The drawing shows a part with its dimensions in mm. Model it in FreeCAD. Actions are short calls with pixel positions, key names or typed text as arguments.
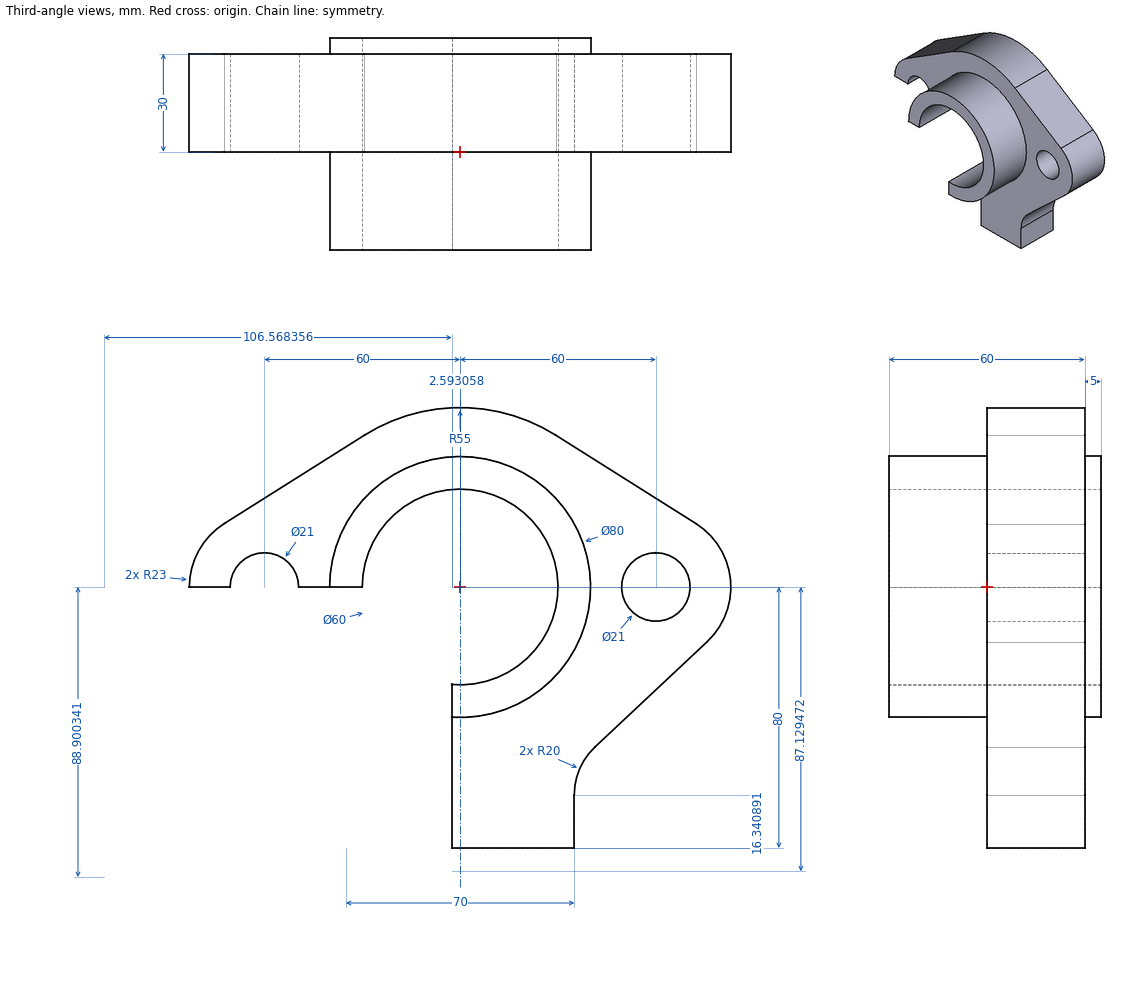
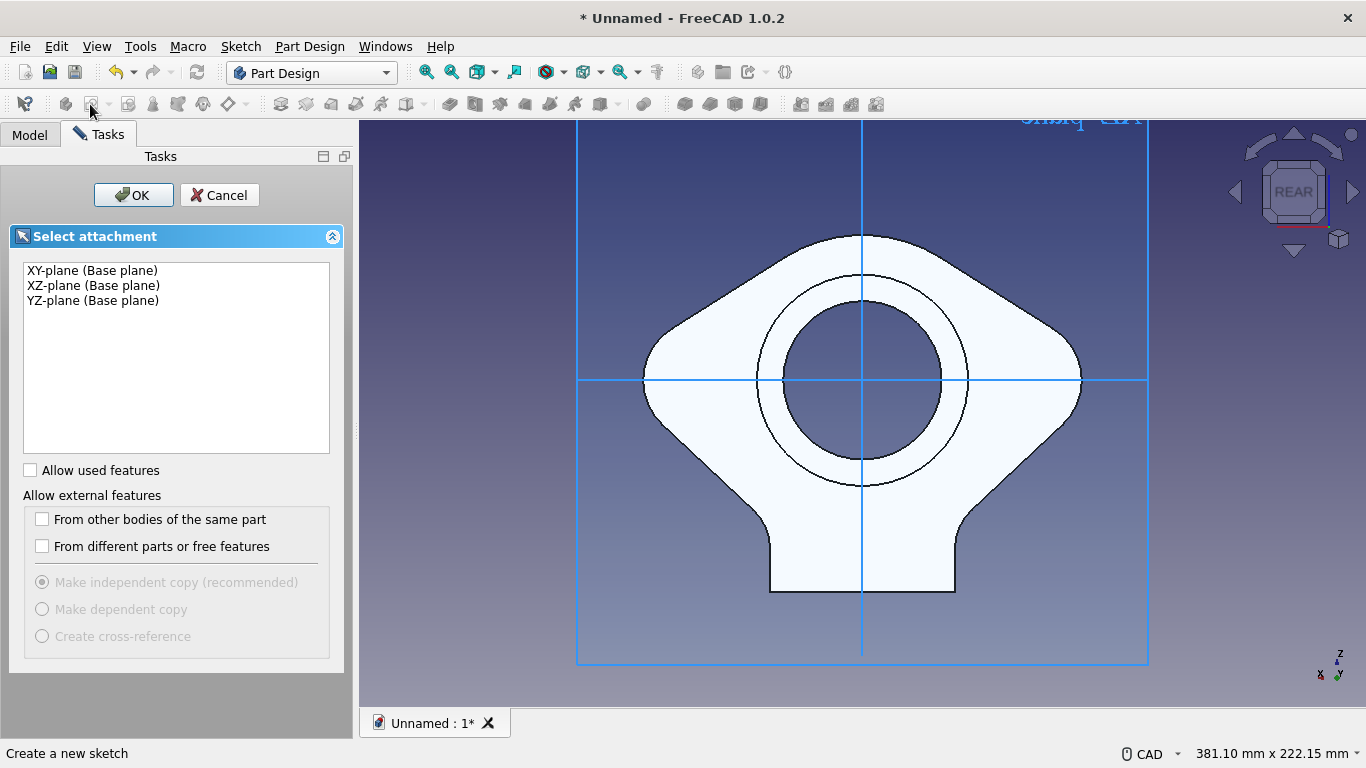
click(84, 286)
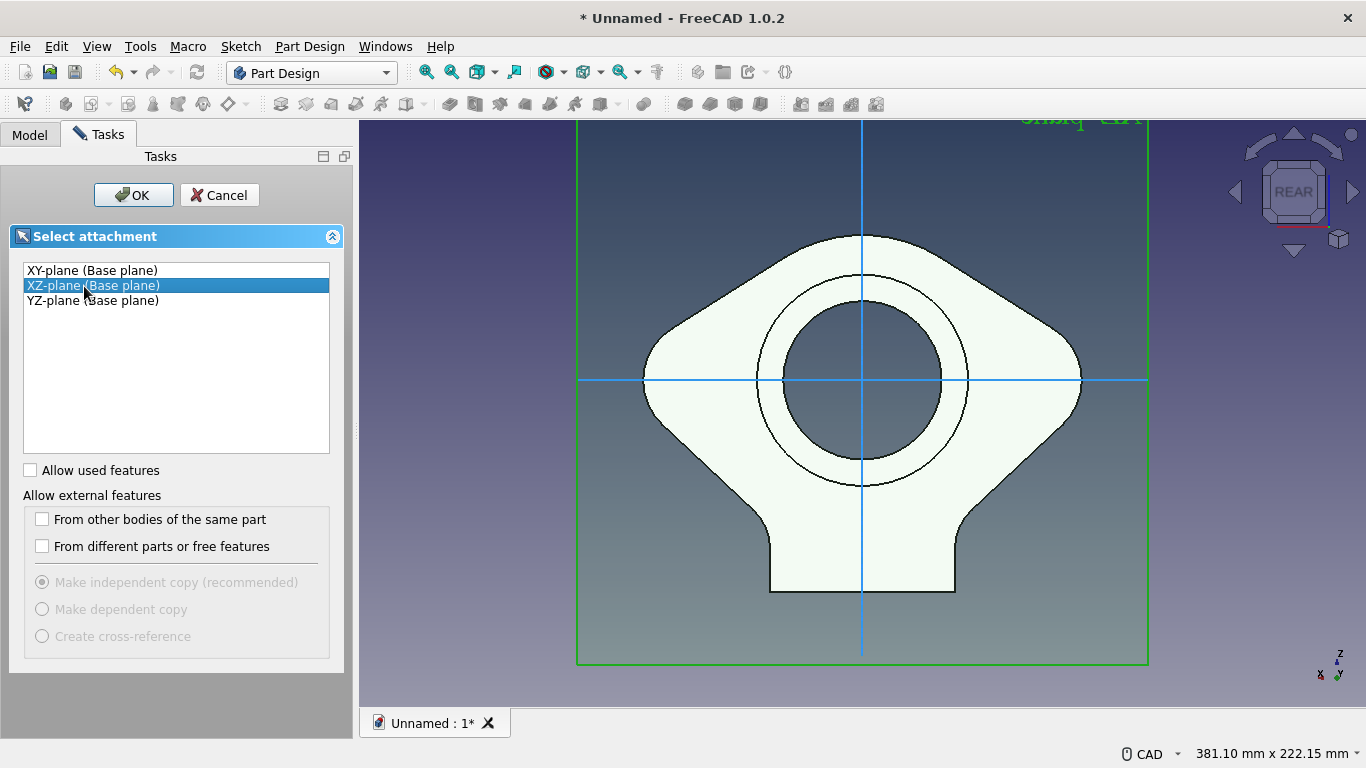
click(134, 195)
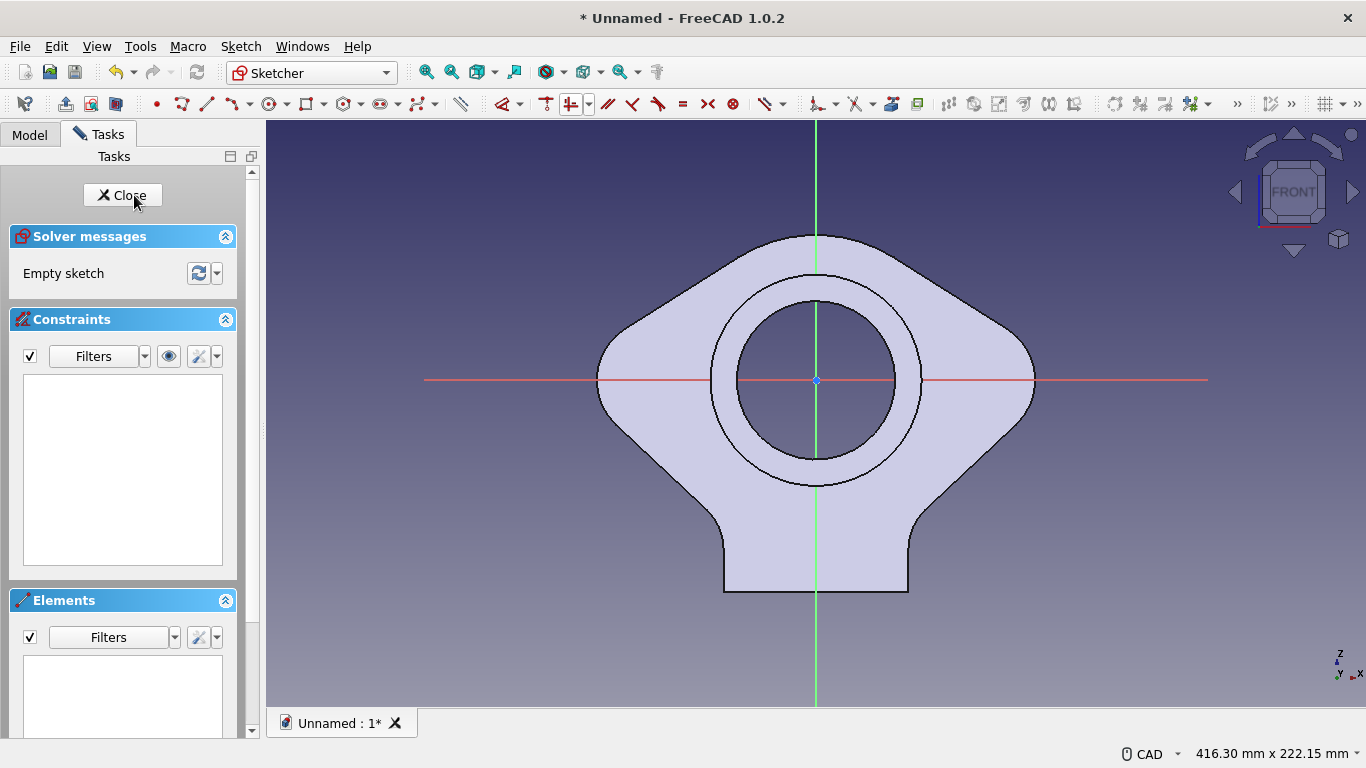
click(116, 104)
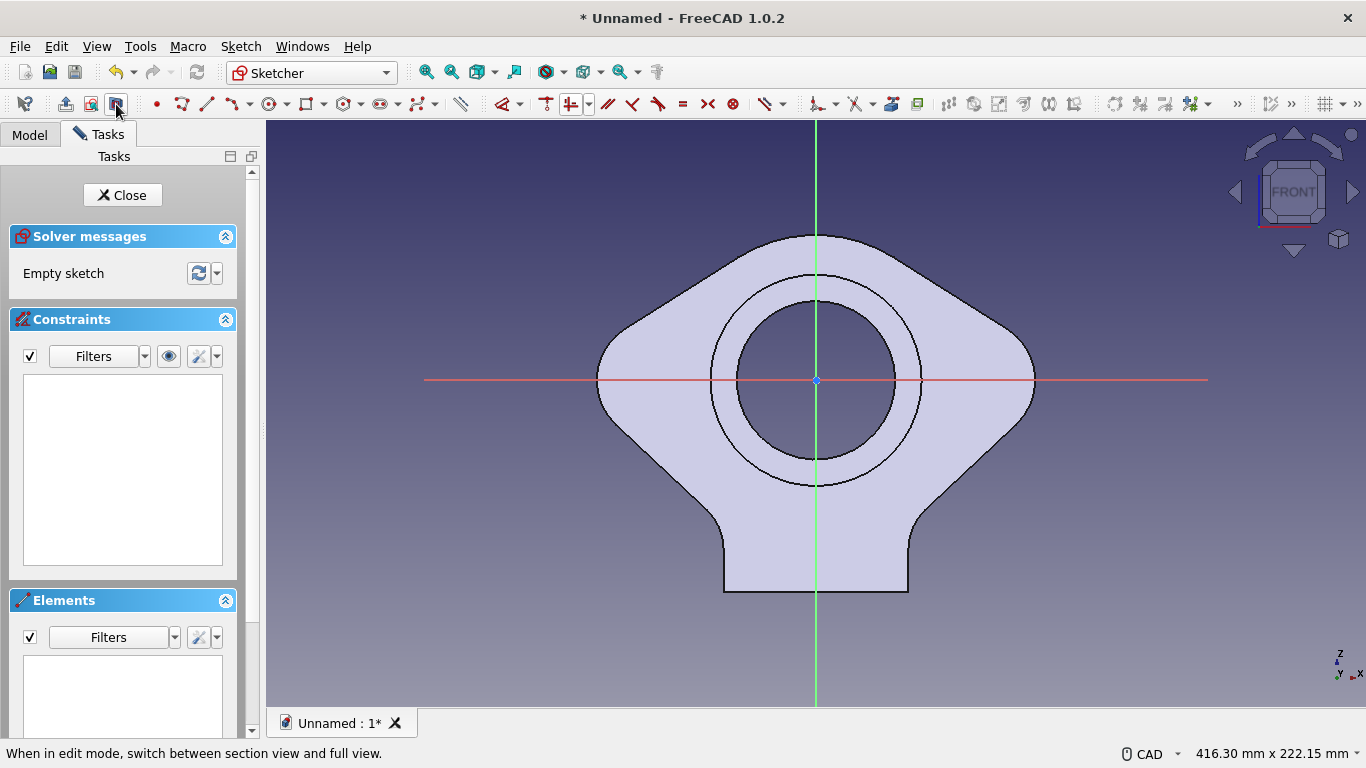
scroll(518, 669, up, 2)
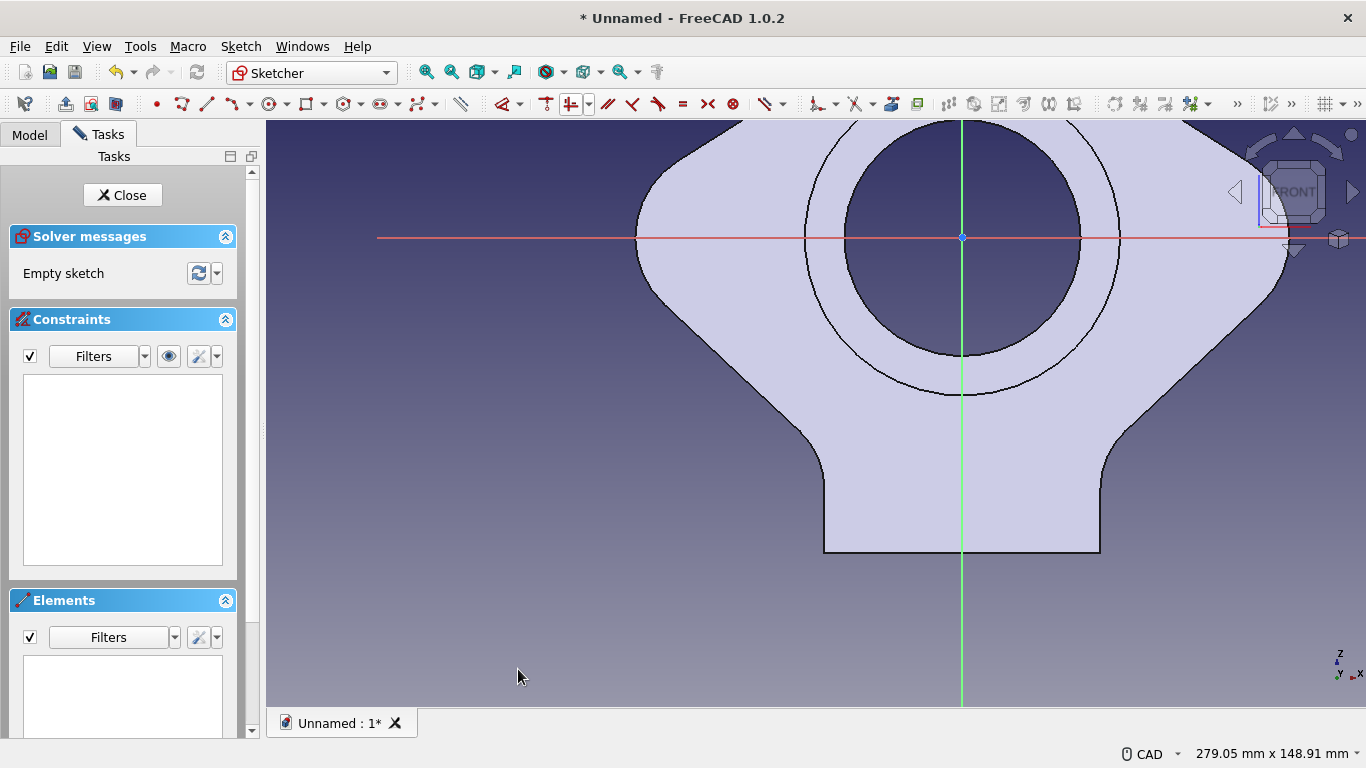
click(182, 104)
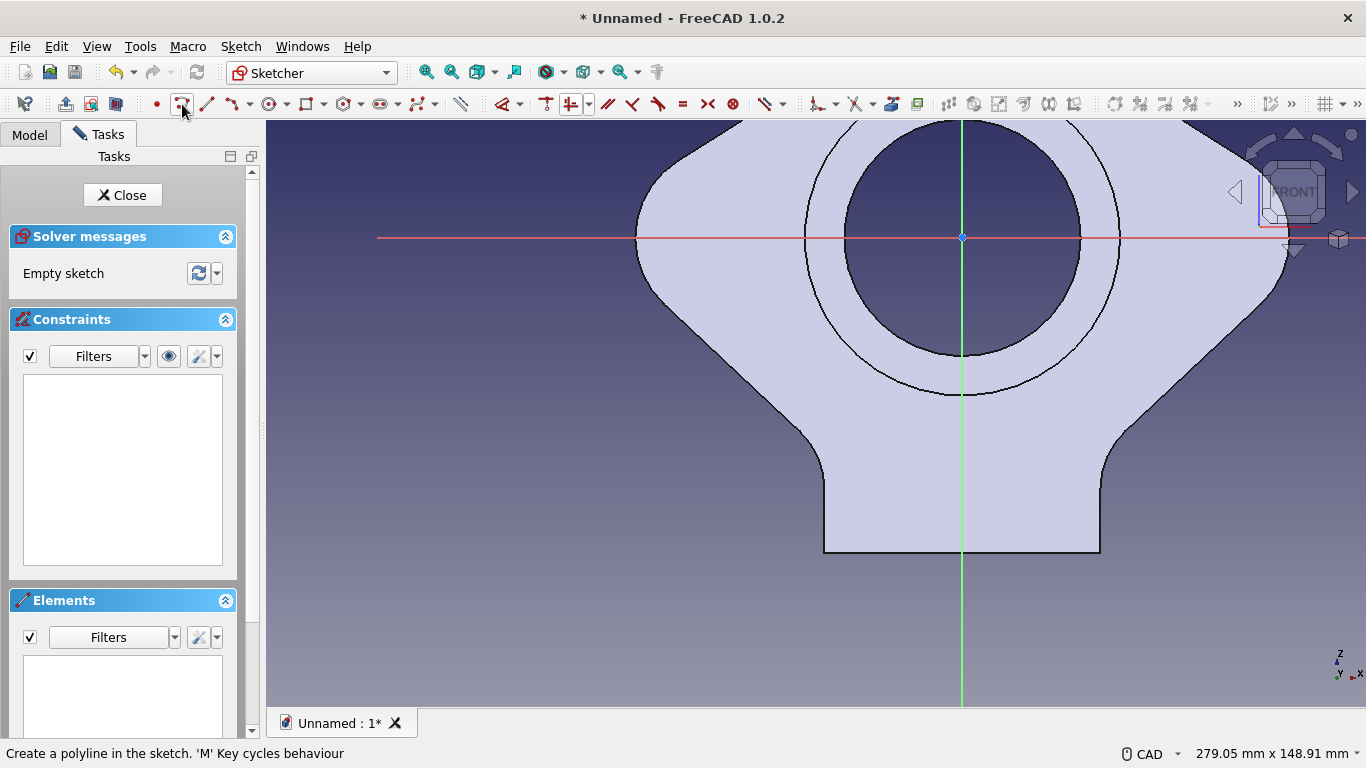
scroll(952, 238, up, 3)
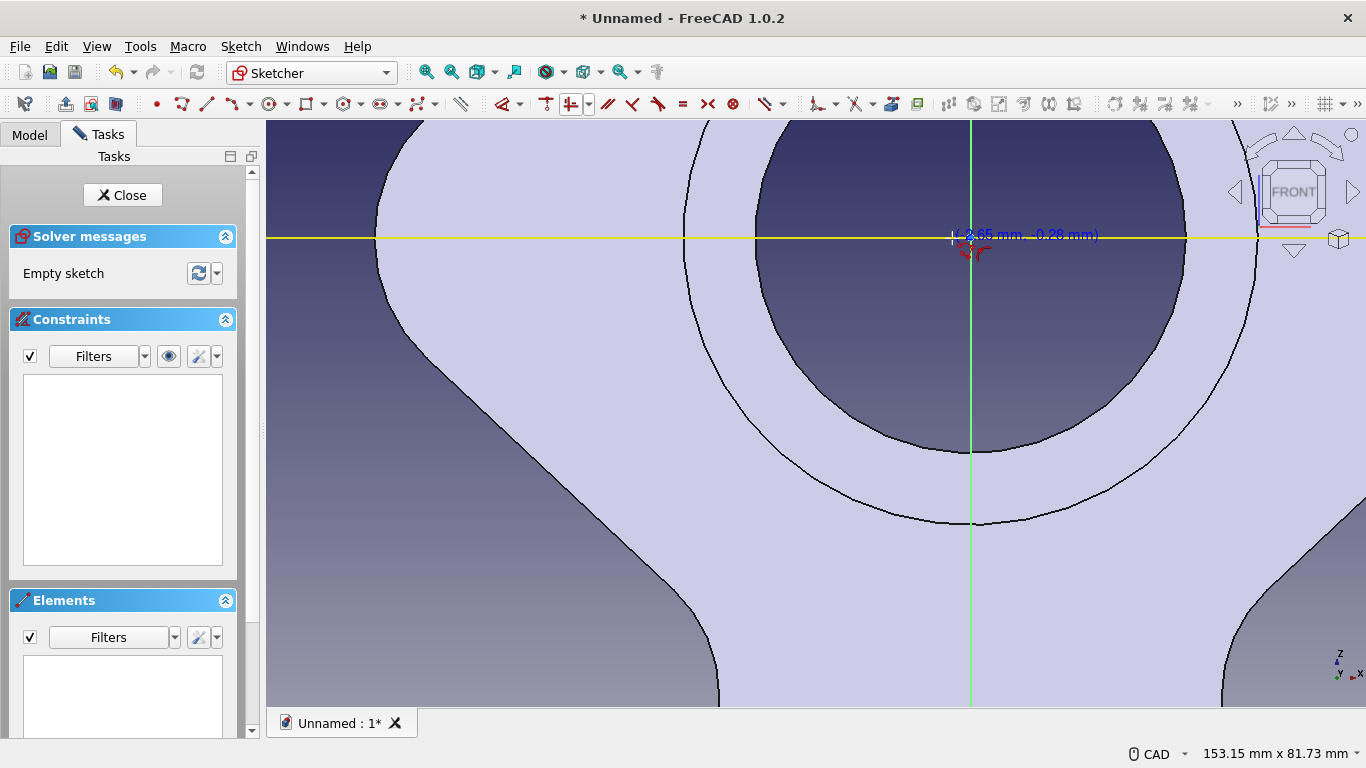
click(952, 238)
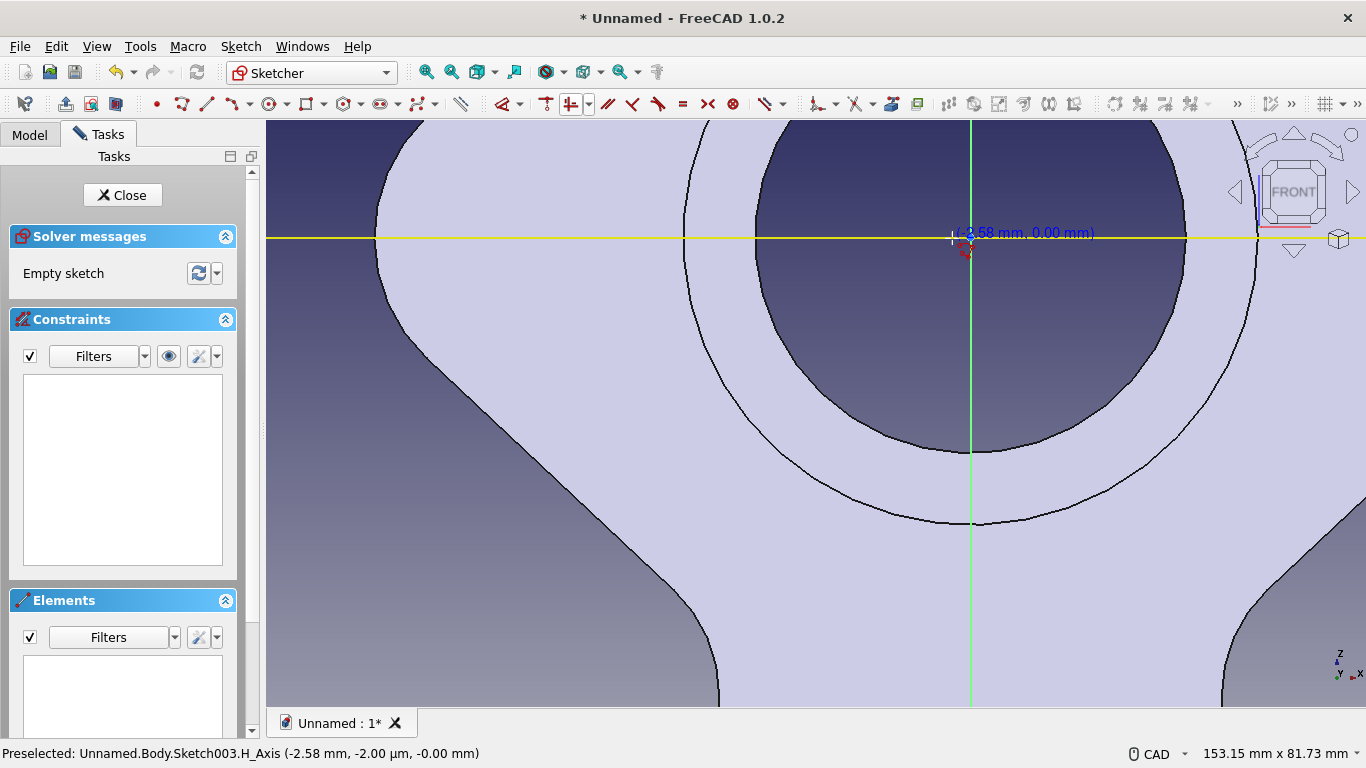
scroll(953, 239, down, 3)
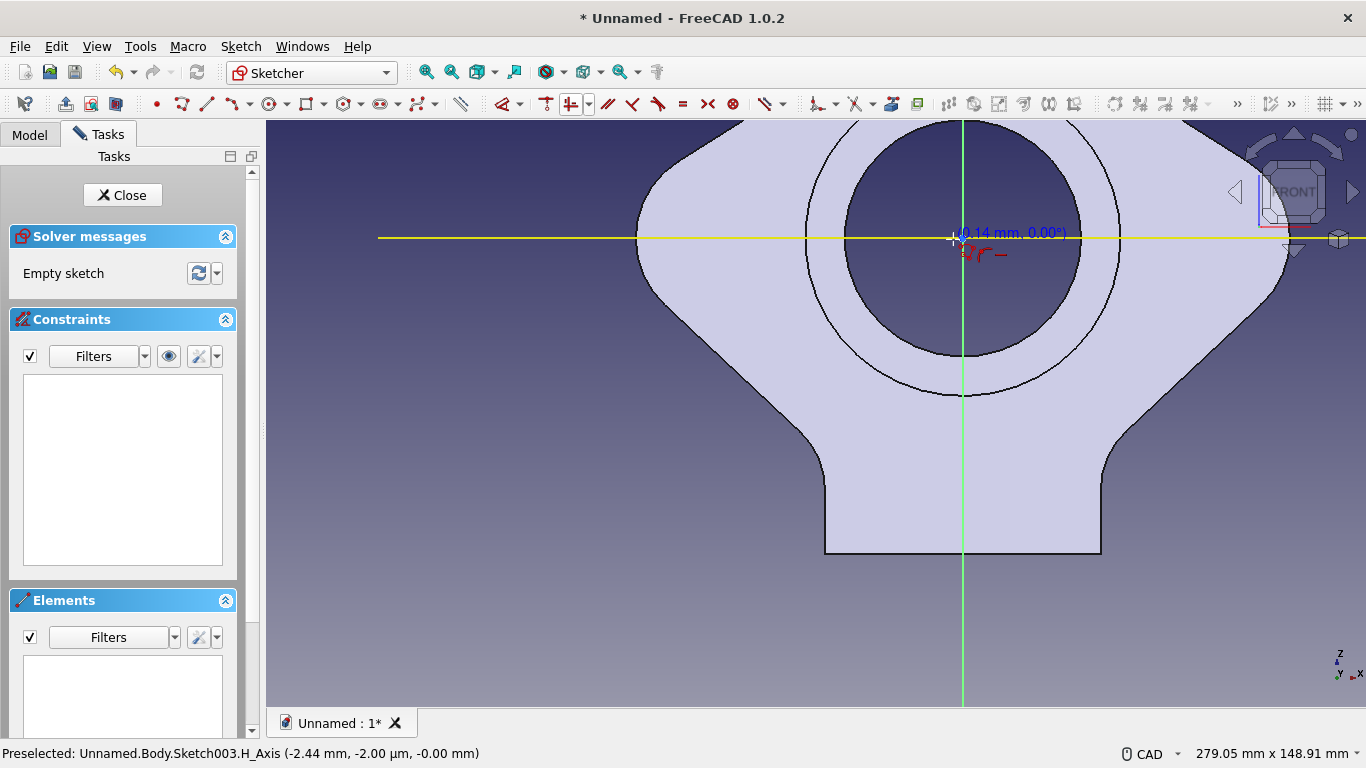
click(533, 247)
click(533, 589)